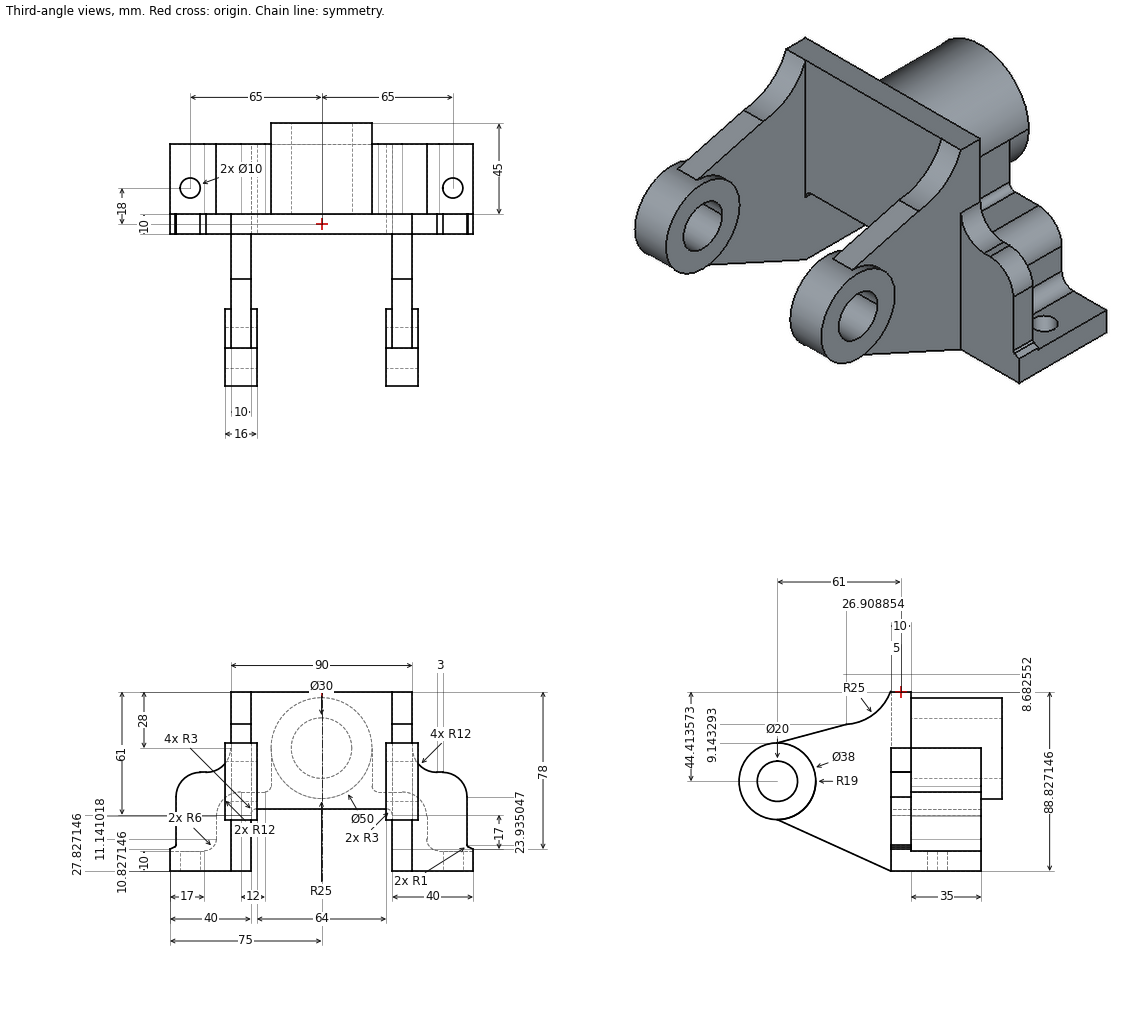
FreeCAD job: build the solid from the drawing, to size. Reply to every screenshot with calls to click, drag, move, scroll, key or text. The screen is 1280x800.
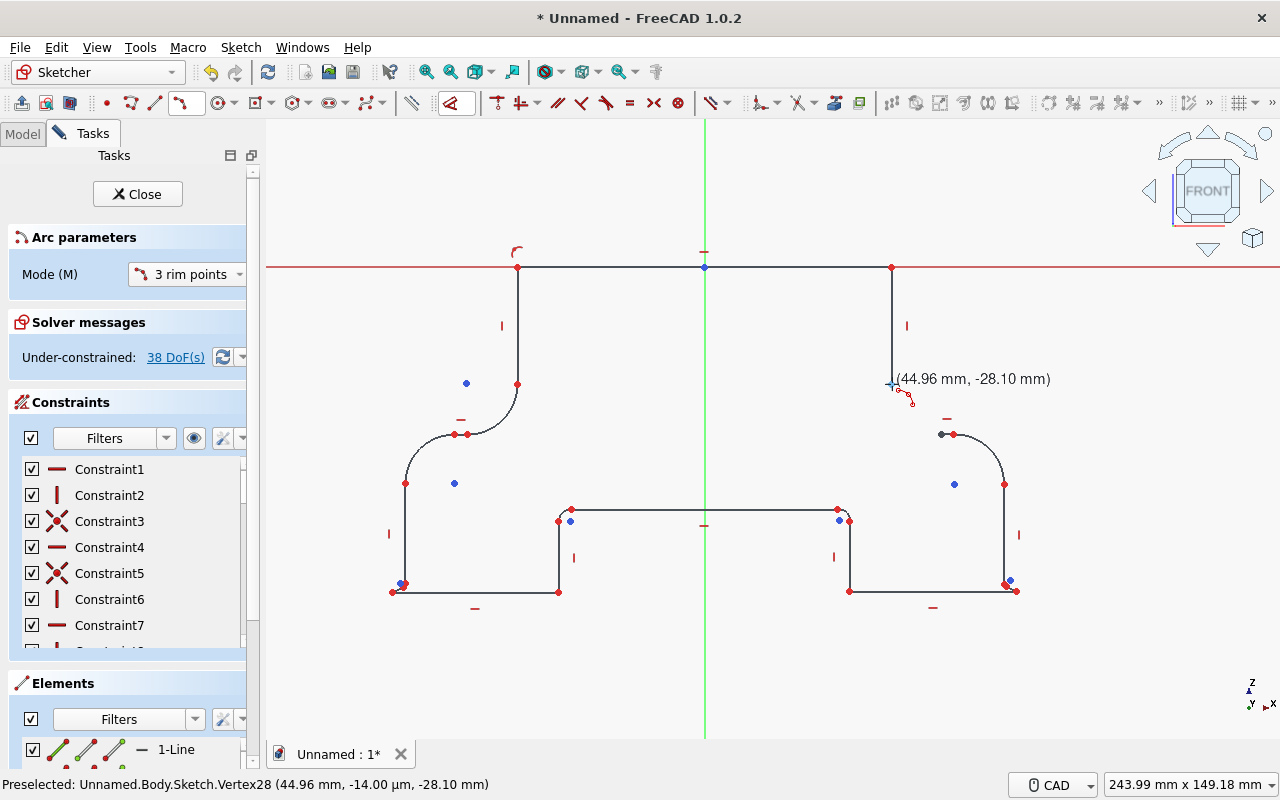
scroll(942, 434, up, 5)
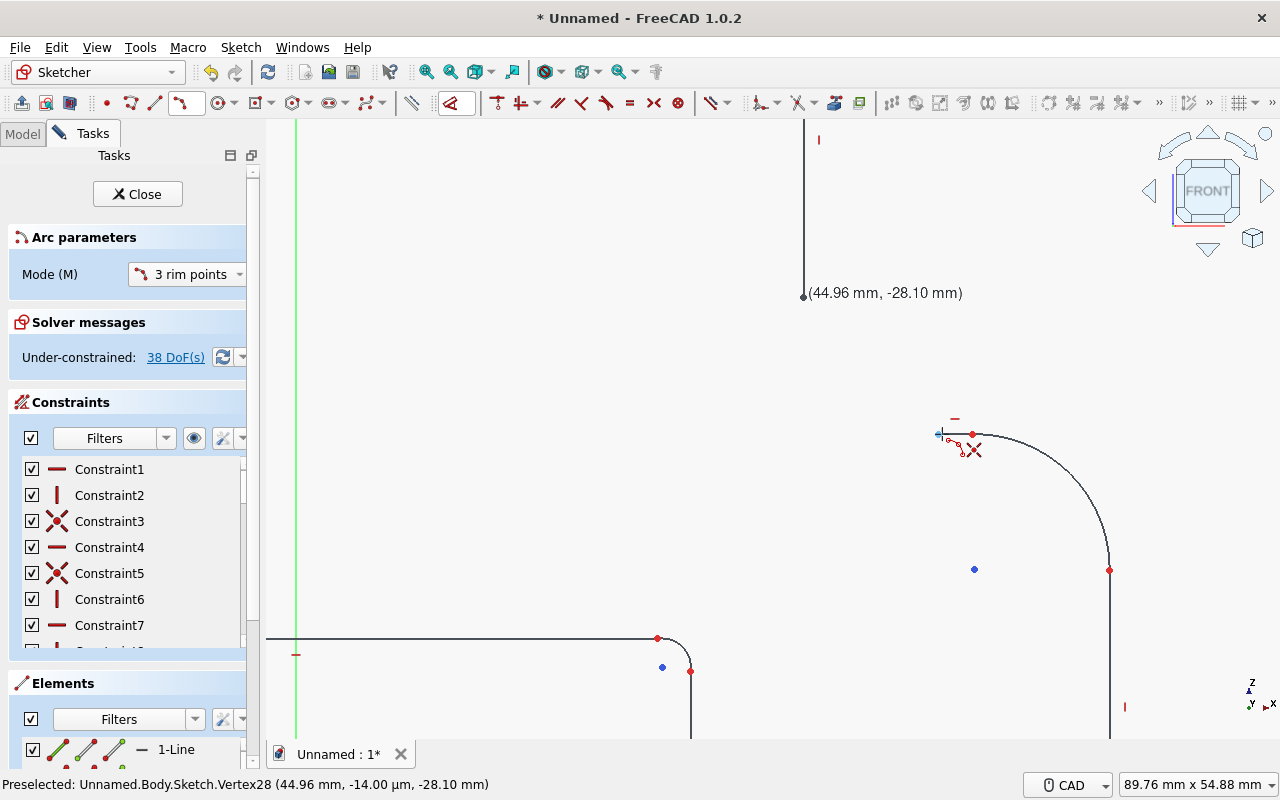
click(939, 434)
click(844, 393)
key(Escape)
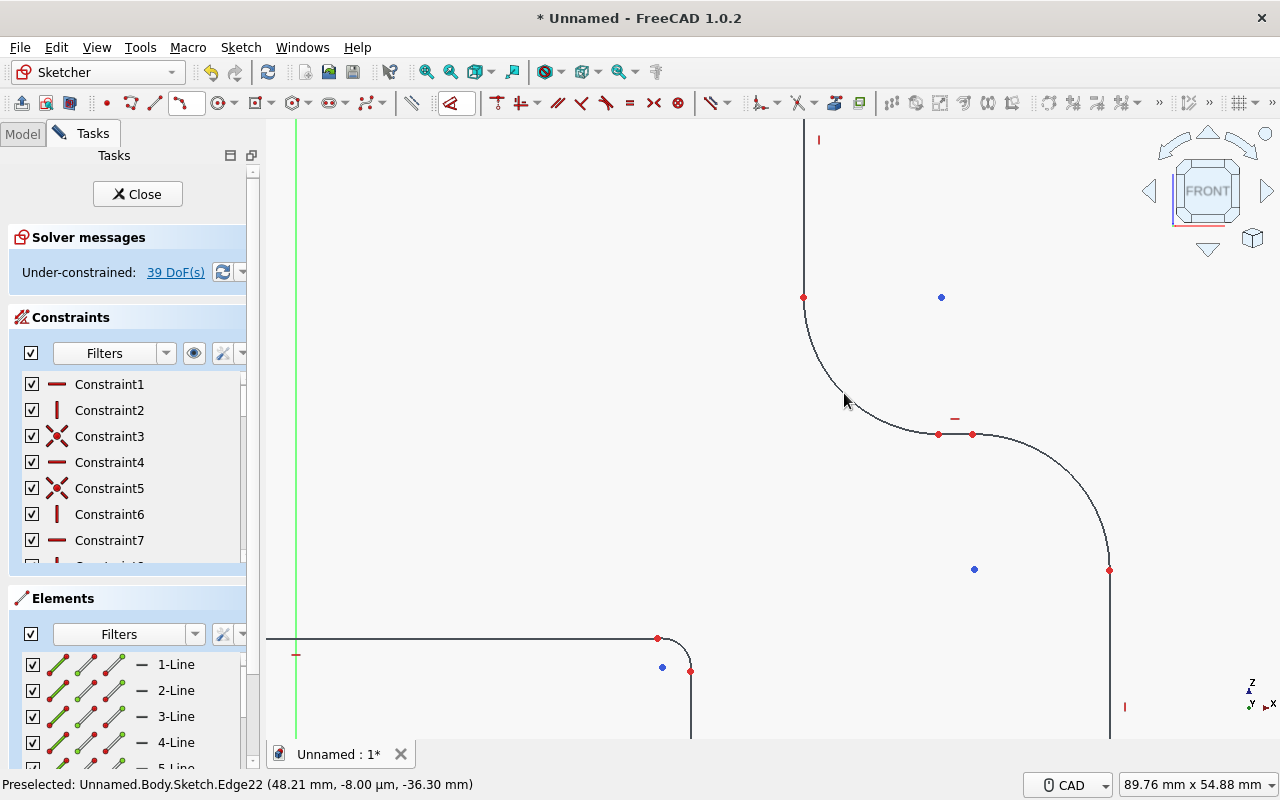
scroll(949, 434, up, 2)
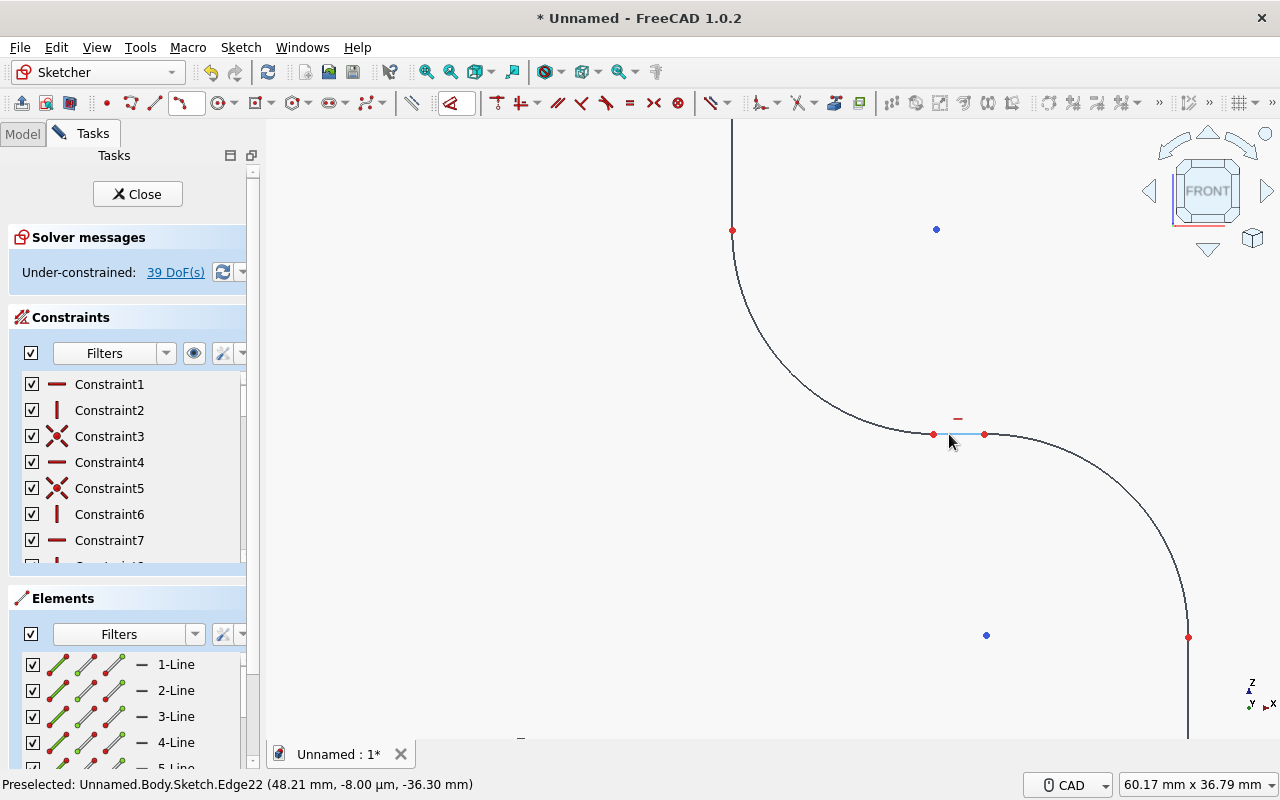
click(949, 434)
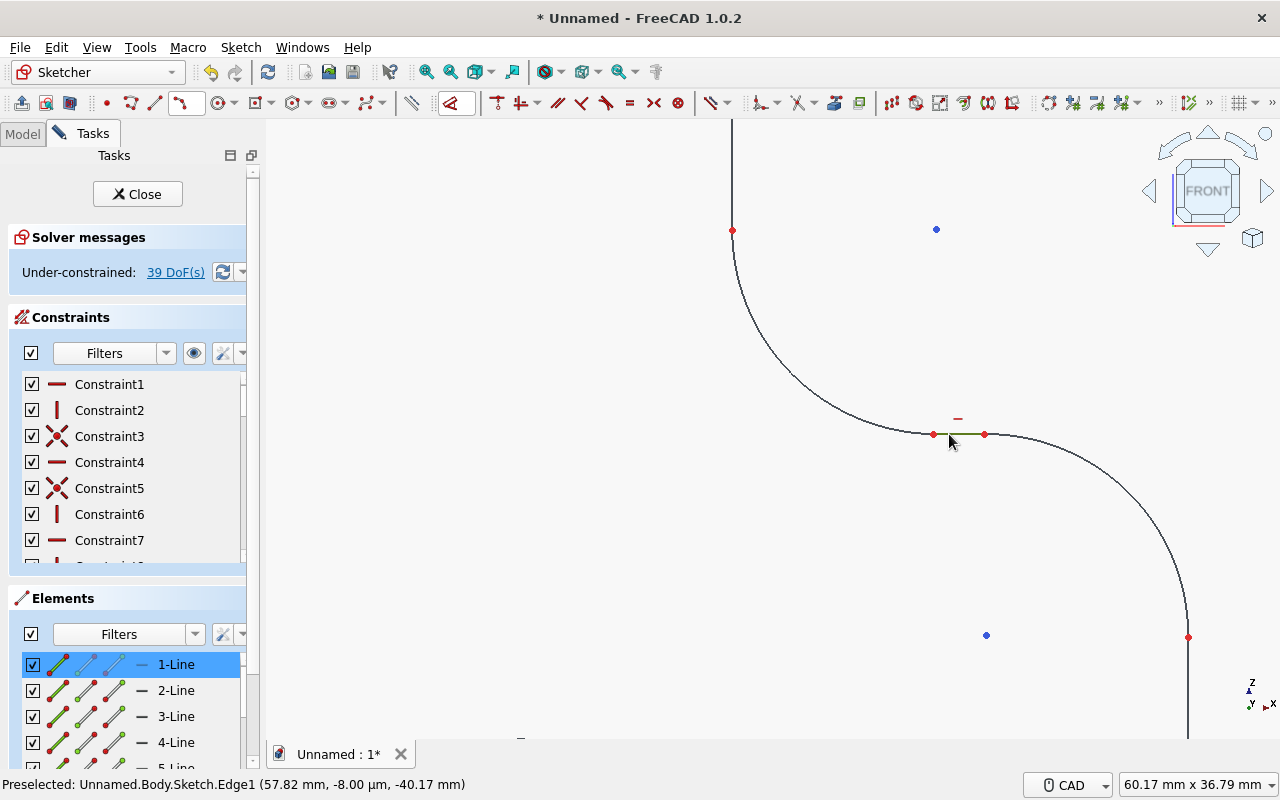
scroll(943, 434, down, 7)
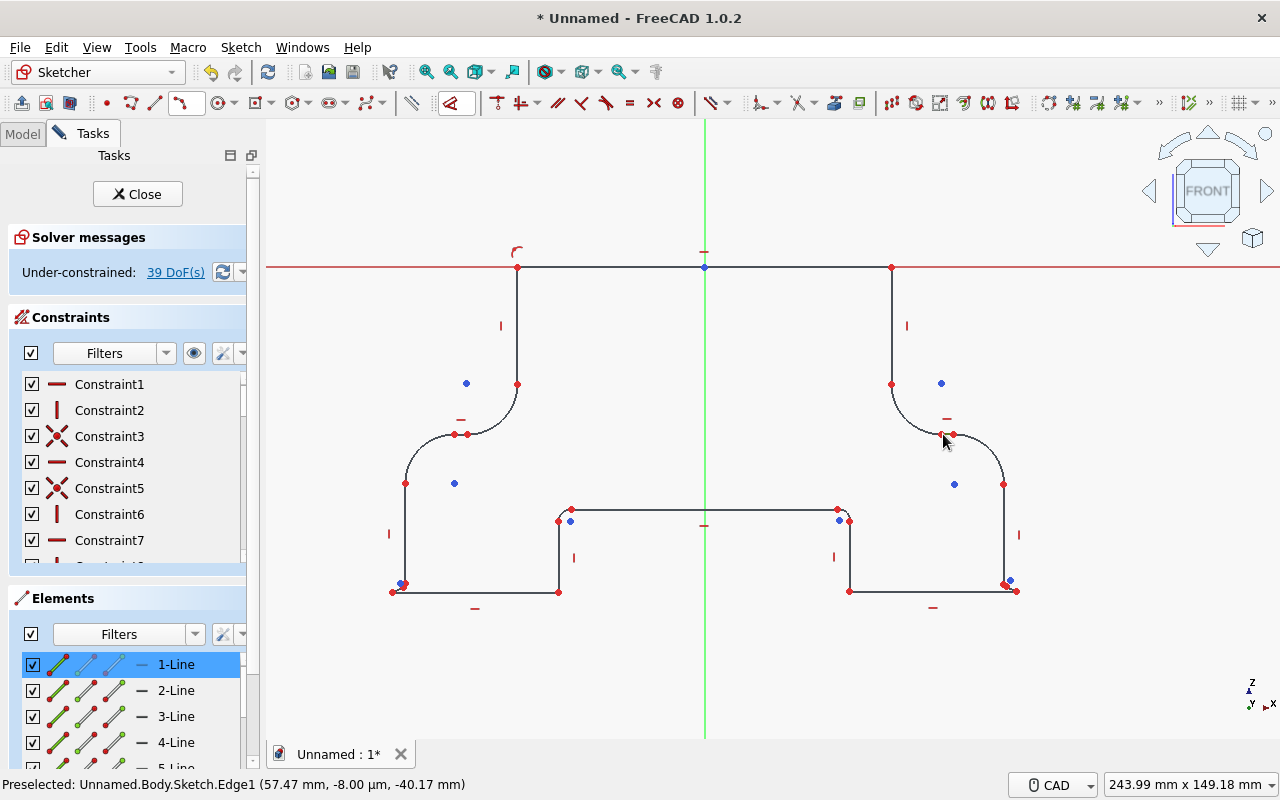
click(977, 440)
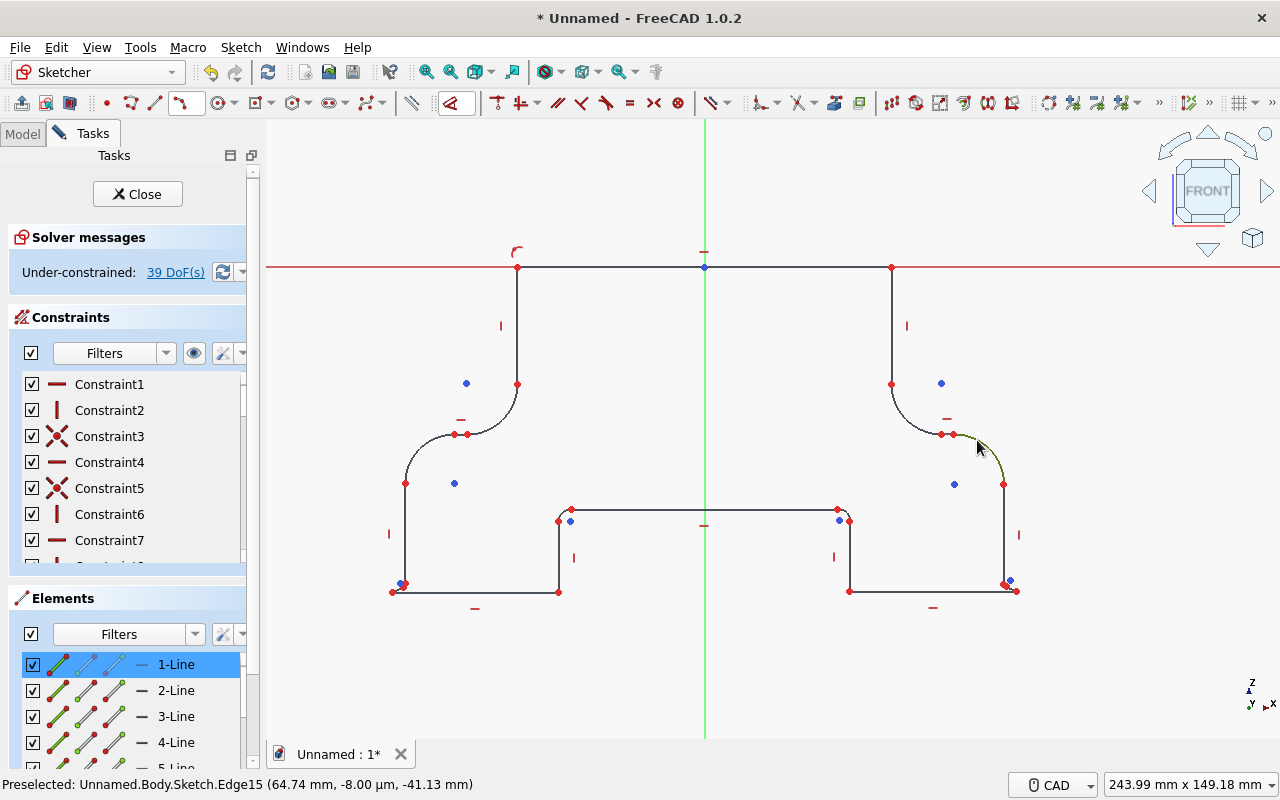
key(t)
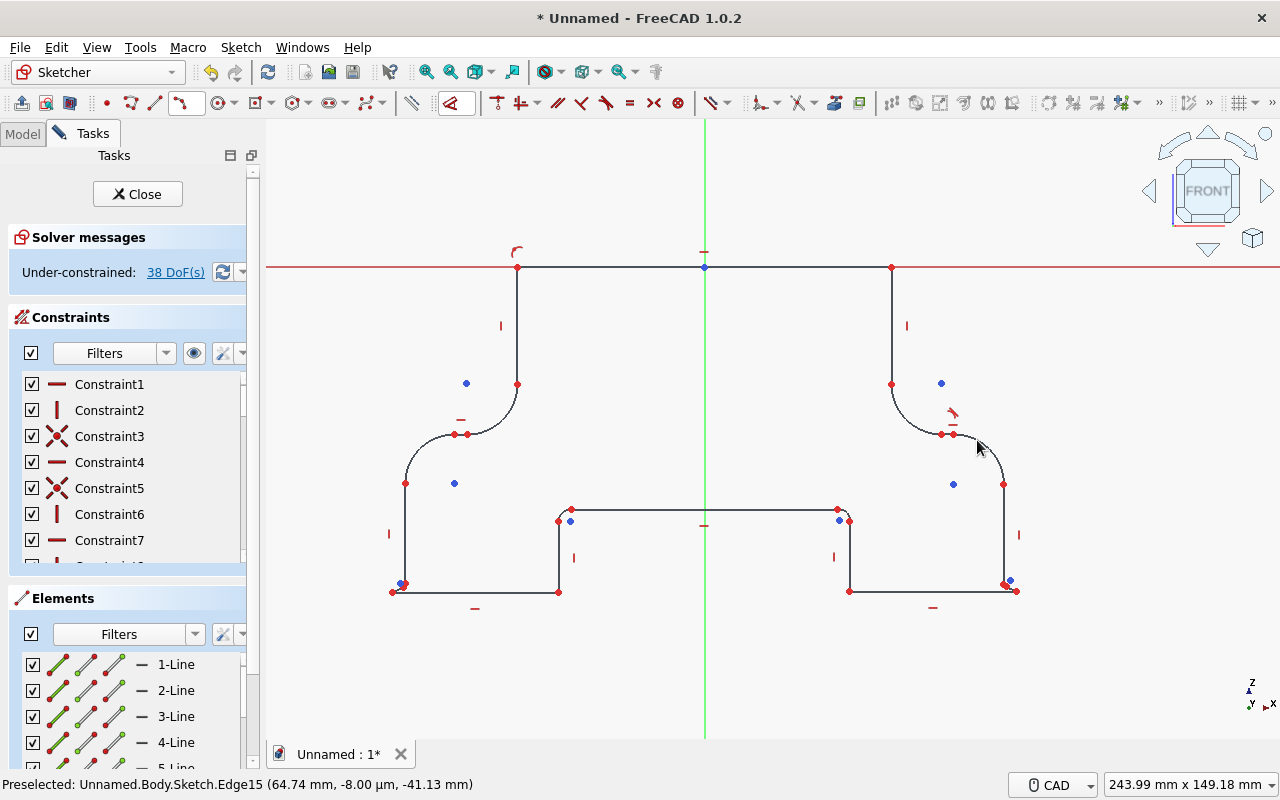
scroll(947, 434, up, 4)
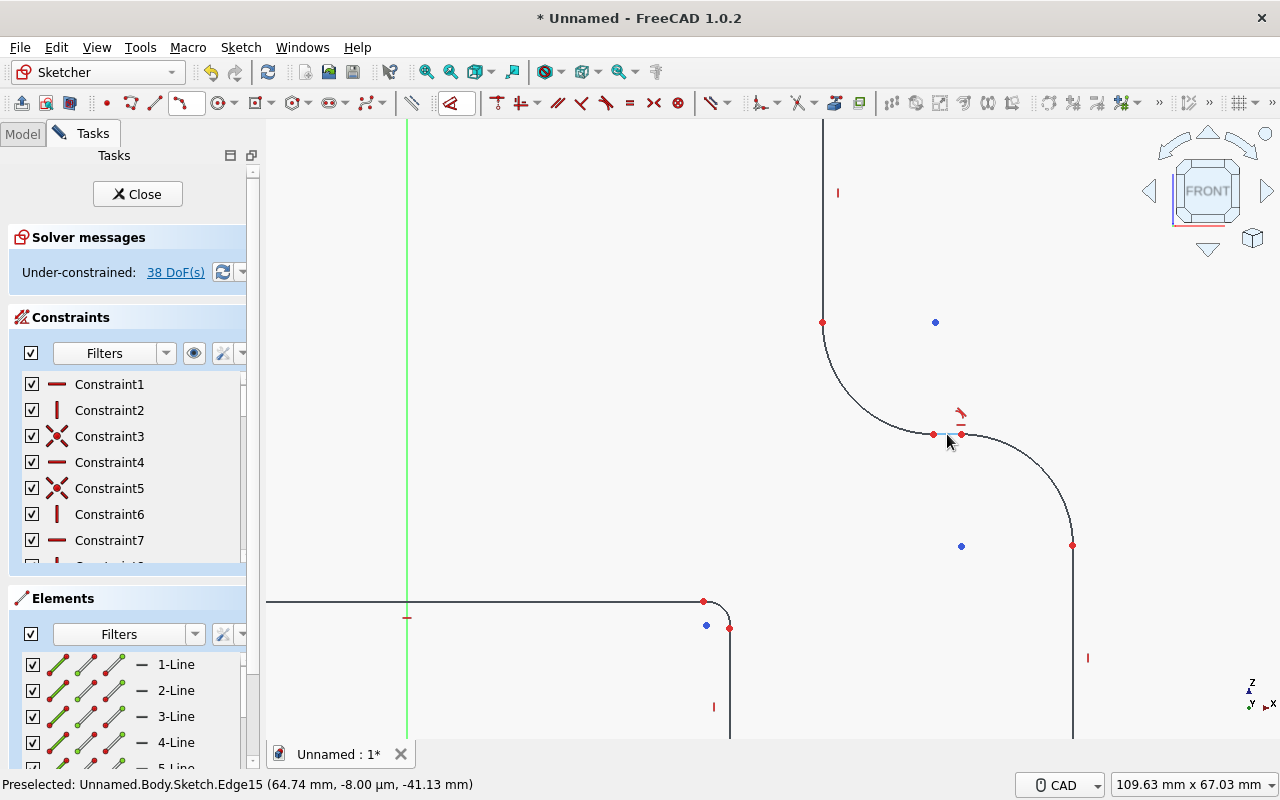
click(947, 434)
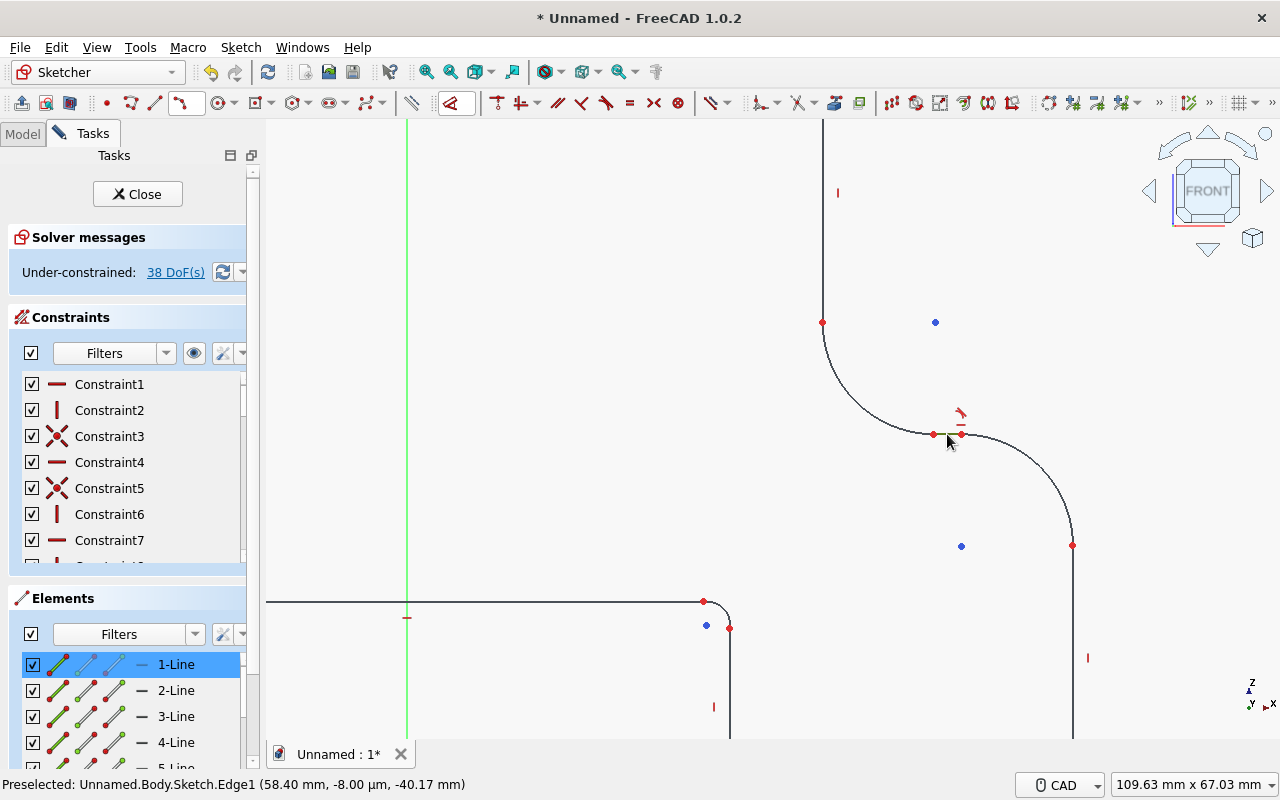
click(835, 373)